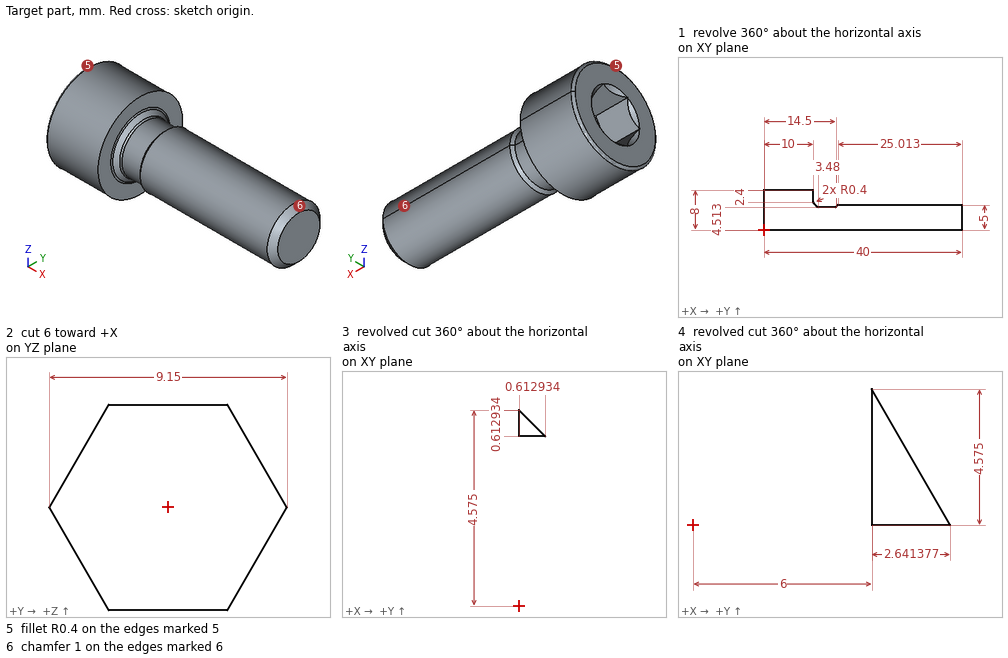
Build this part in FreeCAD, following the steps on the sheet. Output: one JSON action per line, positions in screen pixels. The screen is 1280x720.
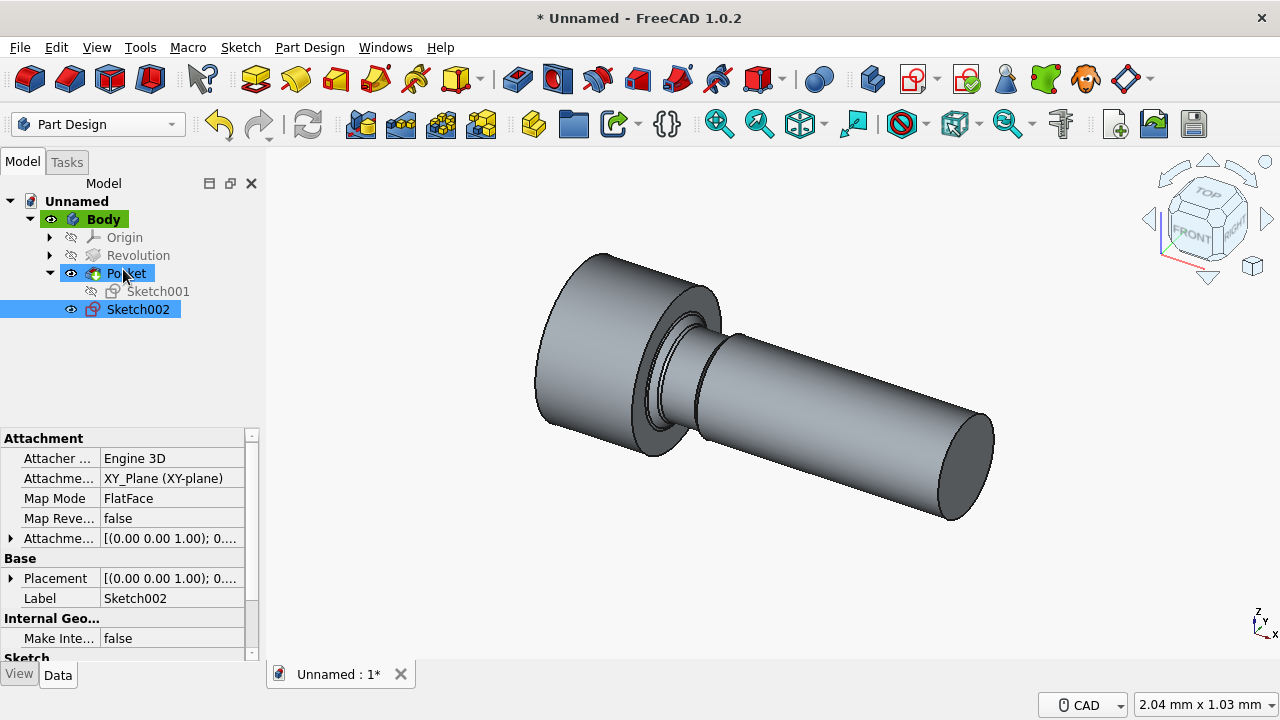
{"action": "left_click", "coordinate": [598, 80]}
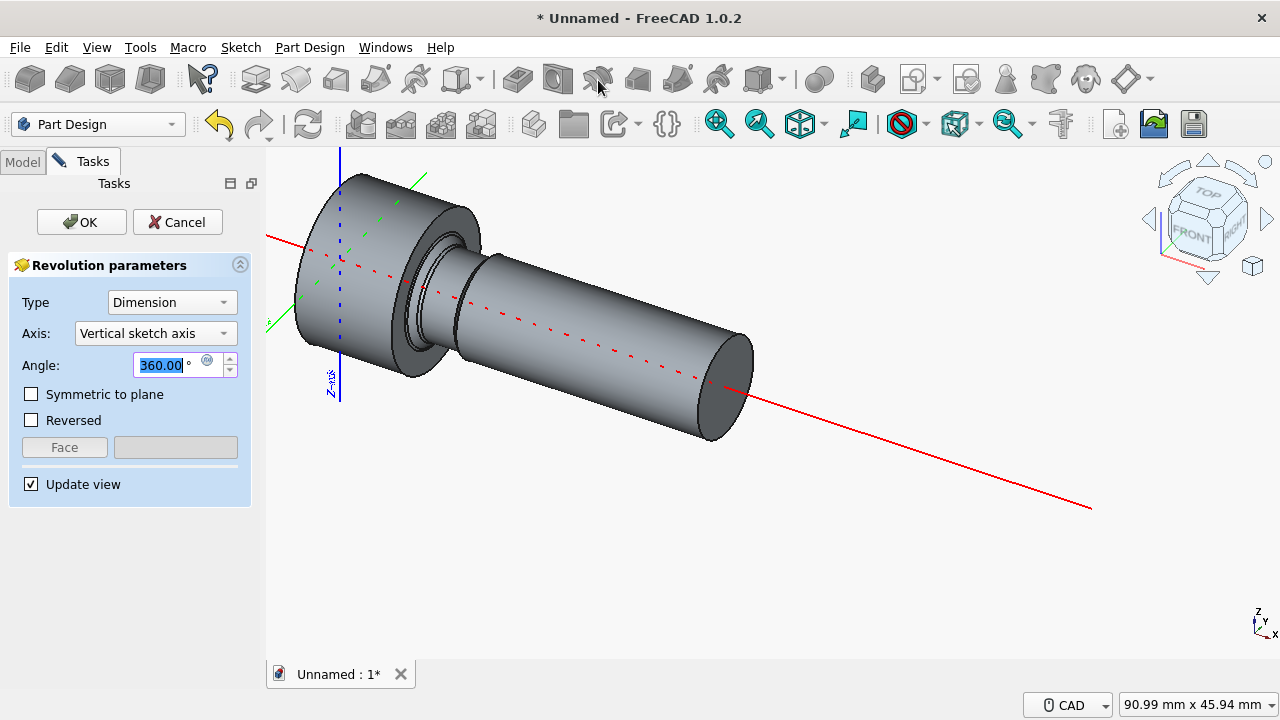
{"action": "left_click", "coordinate": [156, 334]}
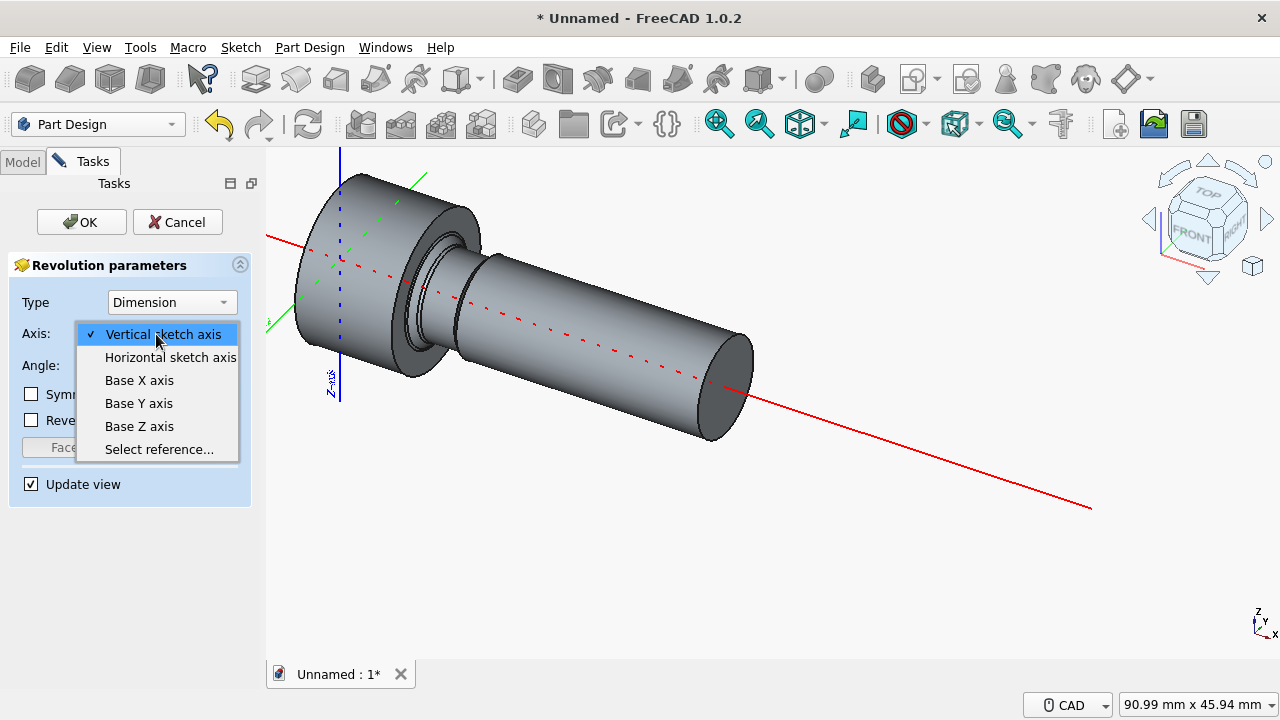
{"action": "left_click", "coordinate": [156, 358]}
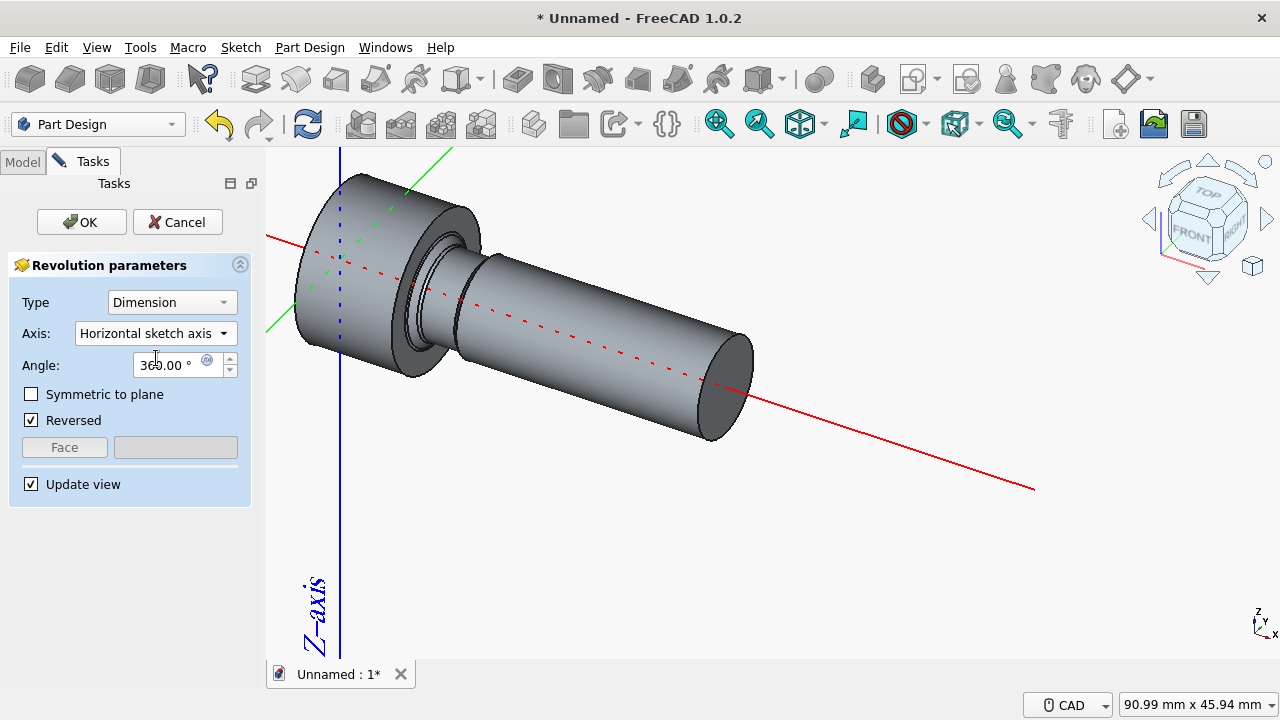
{"action": "left_click", "coordinate": [82, 222]}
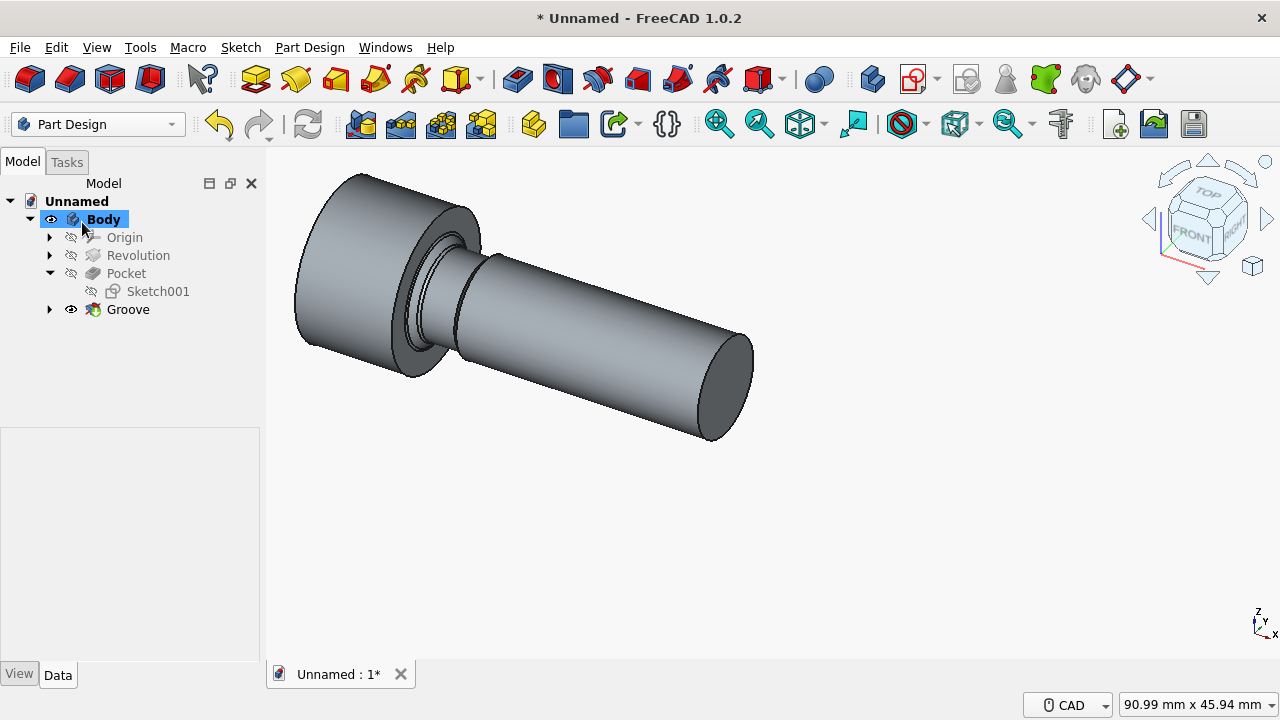
{"action": "left_click", "coordinate": [720, 124]}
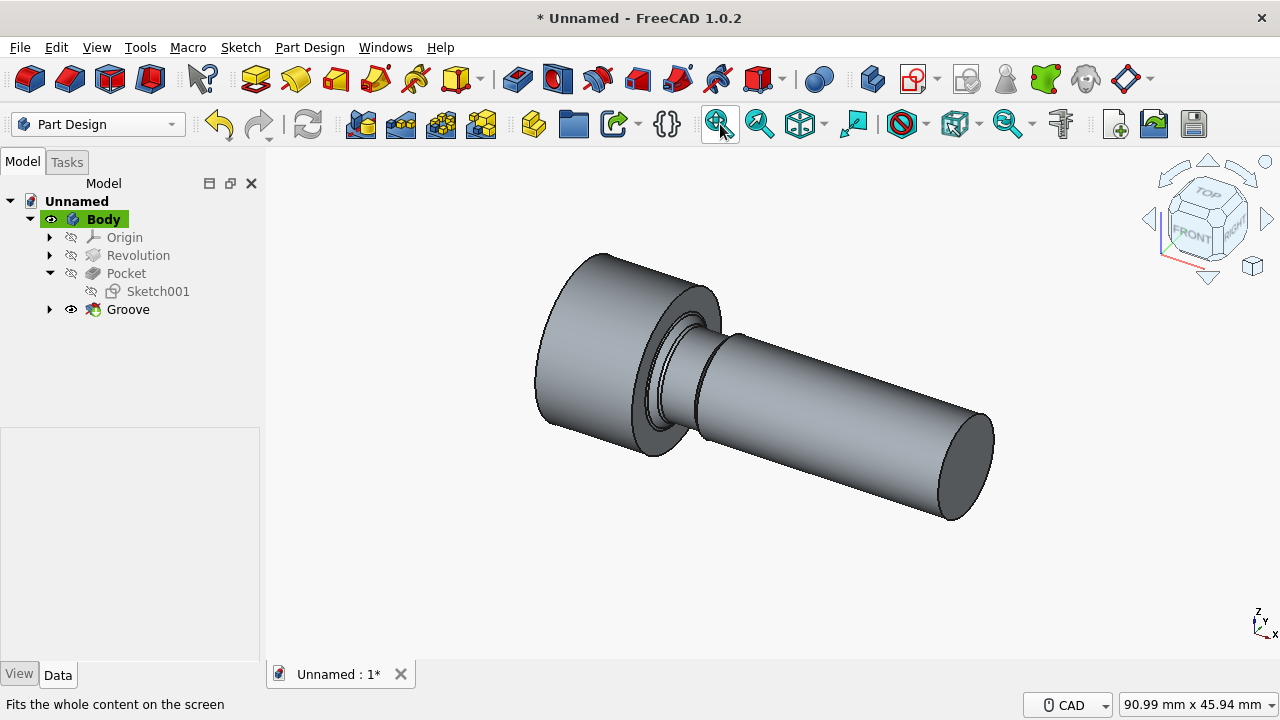
{"action": "left_click", "coordinate": [914, 80]}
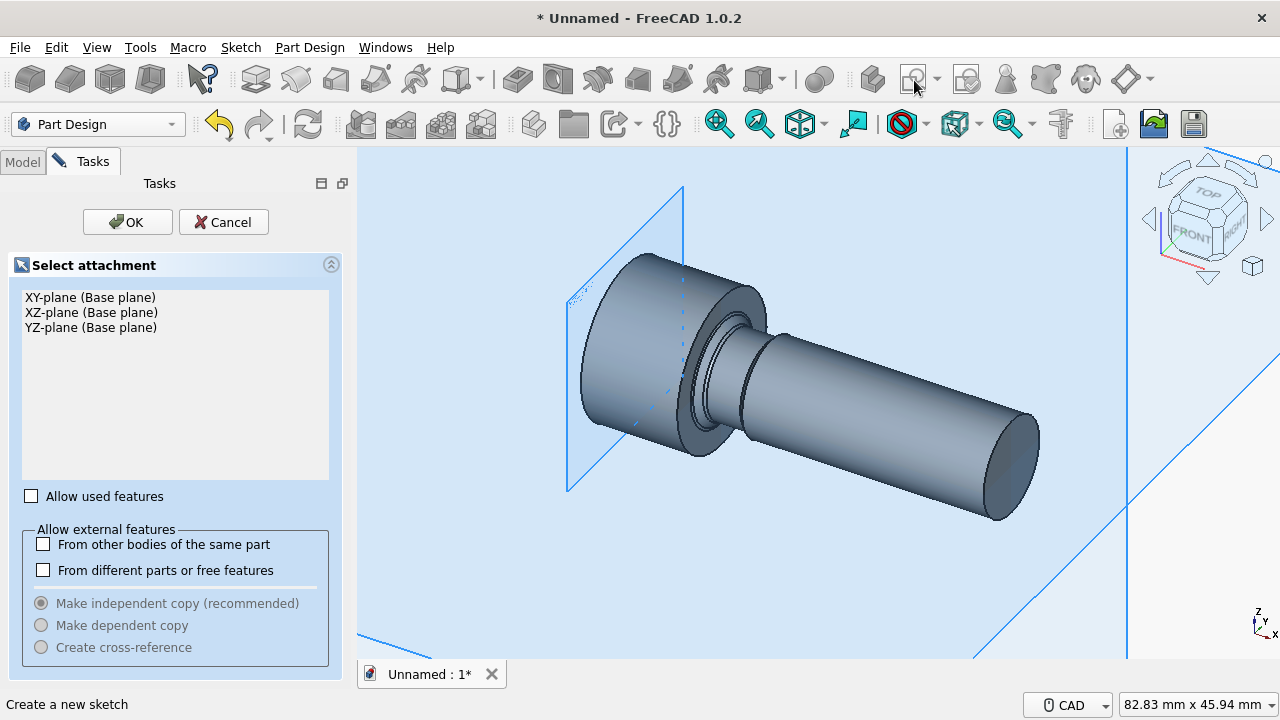
{"action": "left_click", "coordinate": [82, 298]}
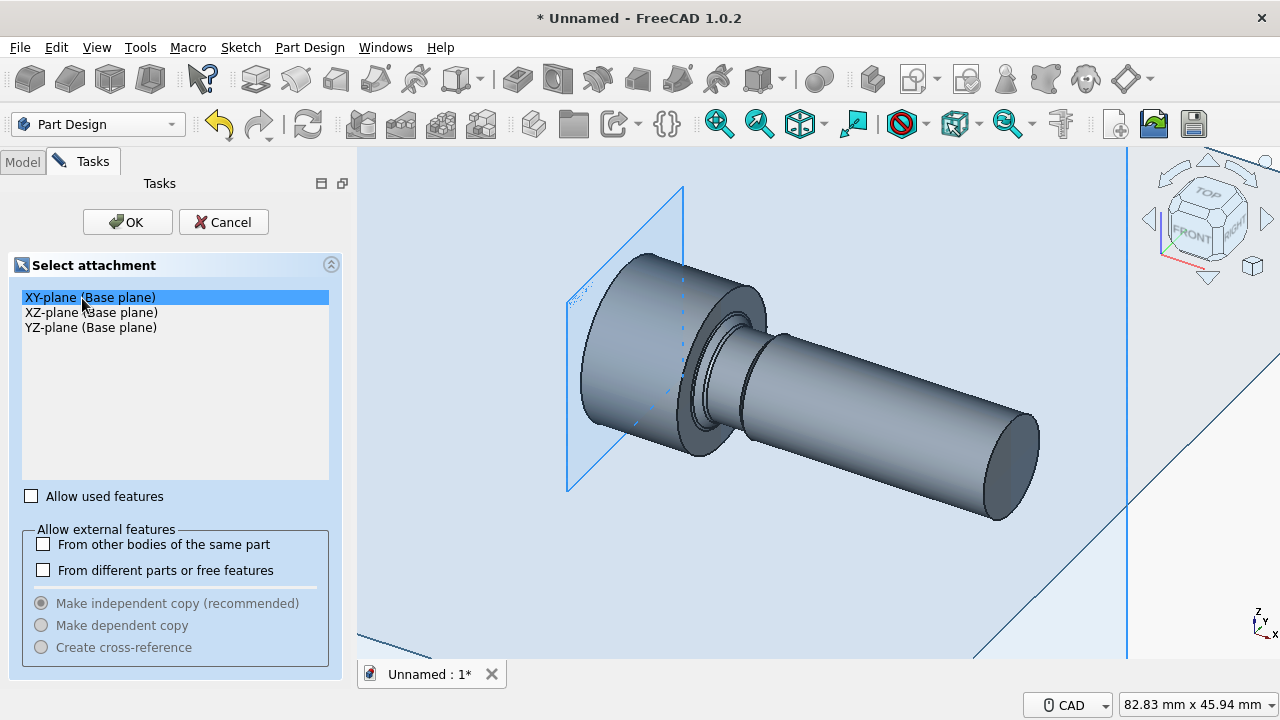
{"action": "left_click", "coordinate": [128, 222]}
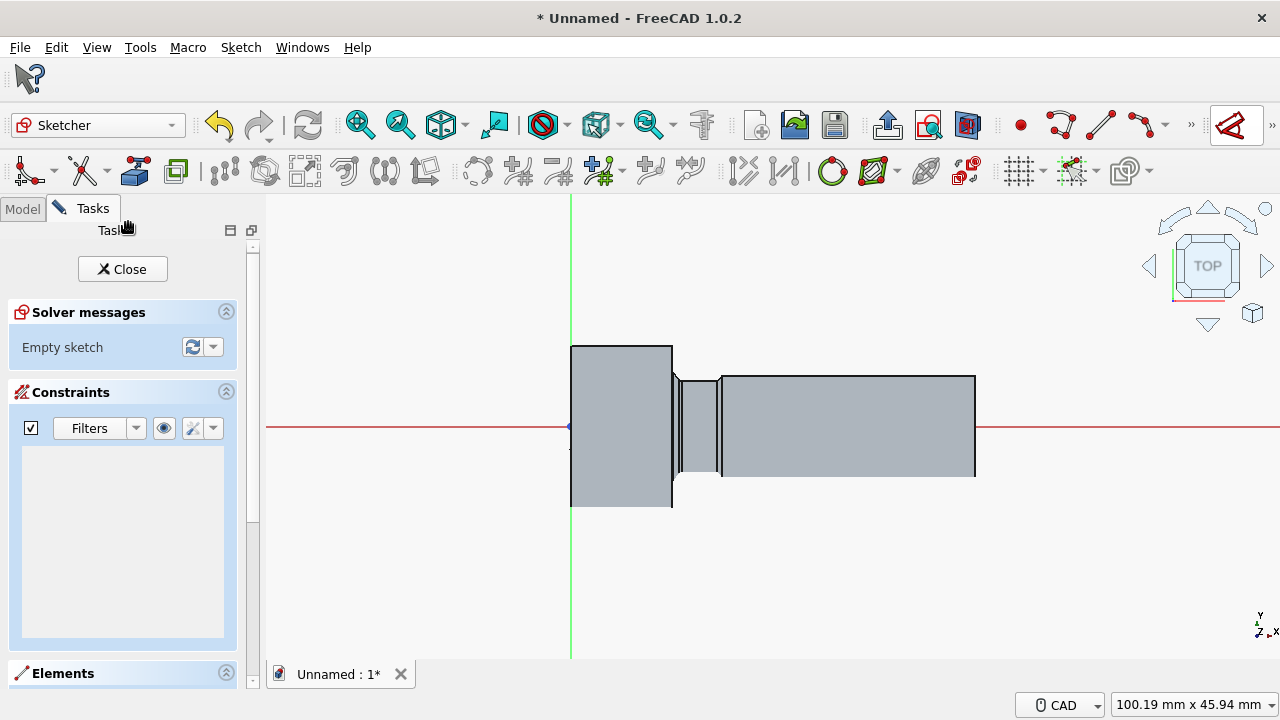
{"action": "key", "text": "q s"}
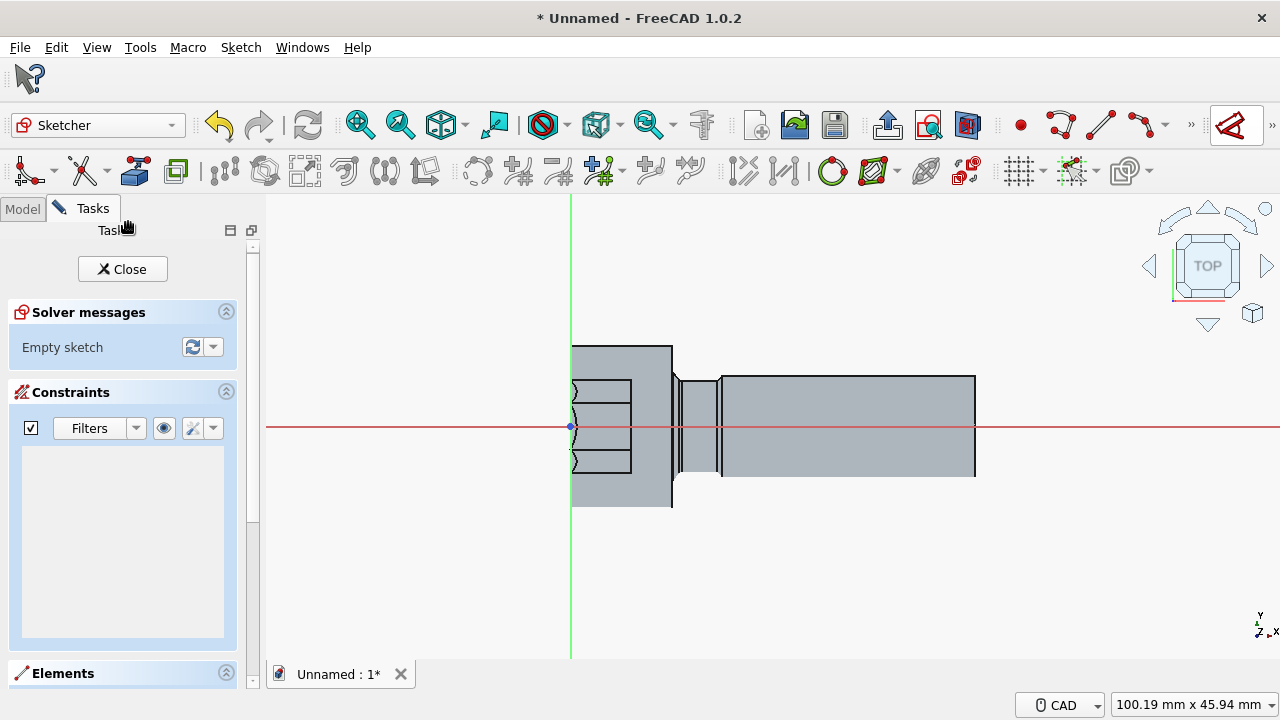
{"action": "scroll", "coordinate": [596, 399], "scroll_direction": "up", "scroll_amount": 9}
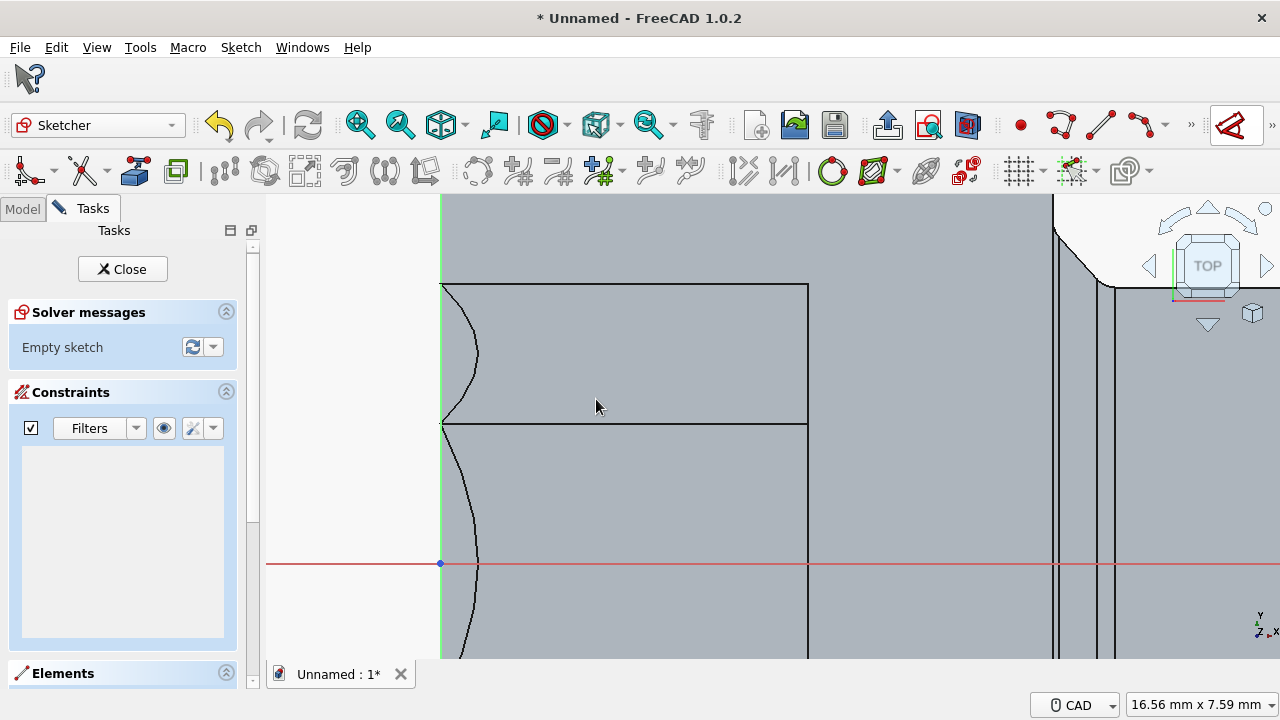
{"action": "left_click", "coordinate": [1062, 126]}